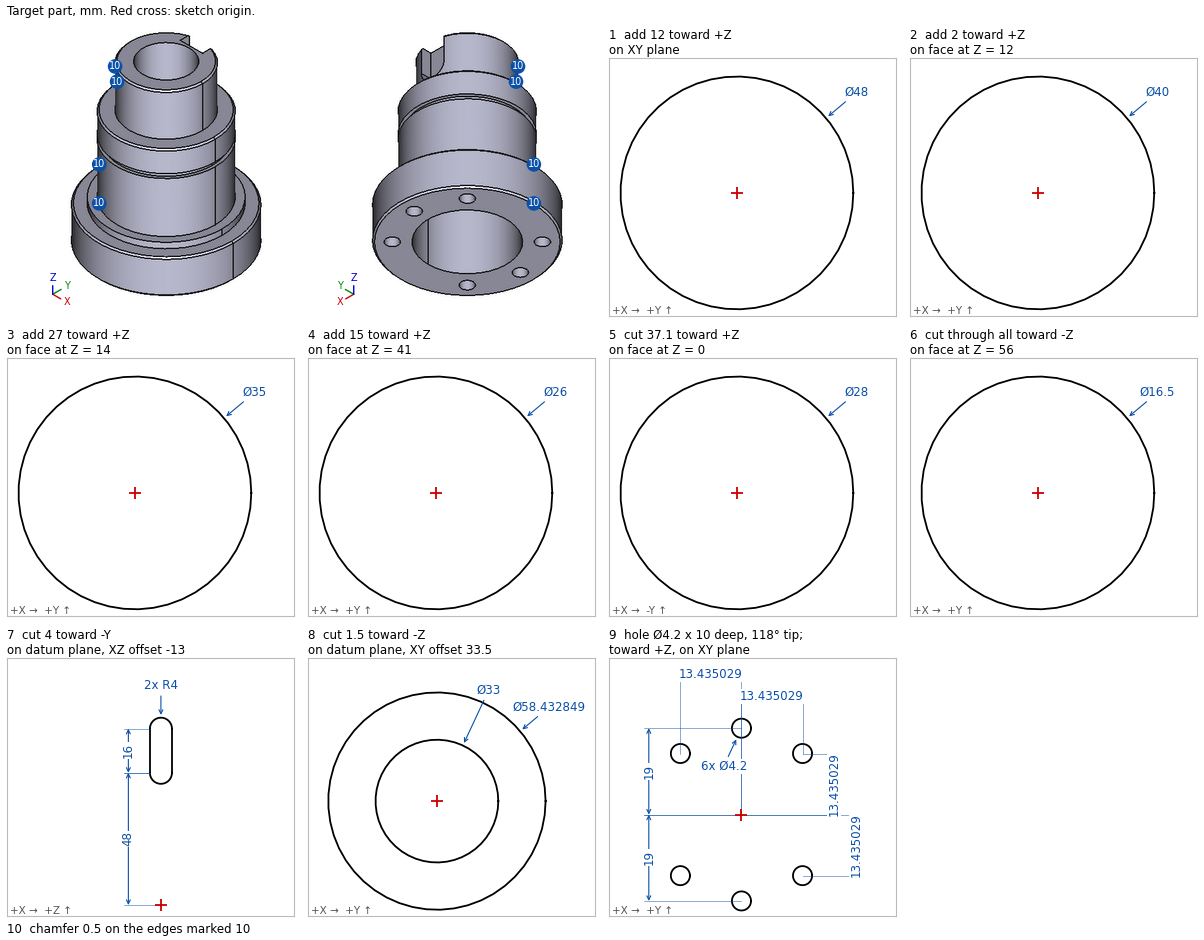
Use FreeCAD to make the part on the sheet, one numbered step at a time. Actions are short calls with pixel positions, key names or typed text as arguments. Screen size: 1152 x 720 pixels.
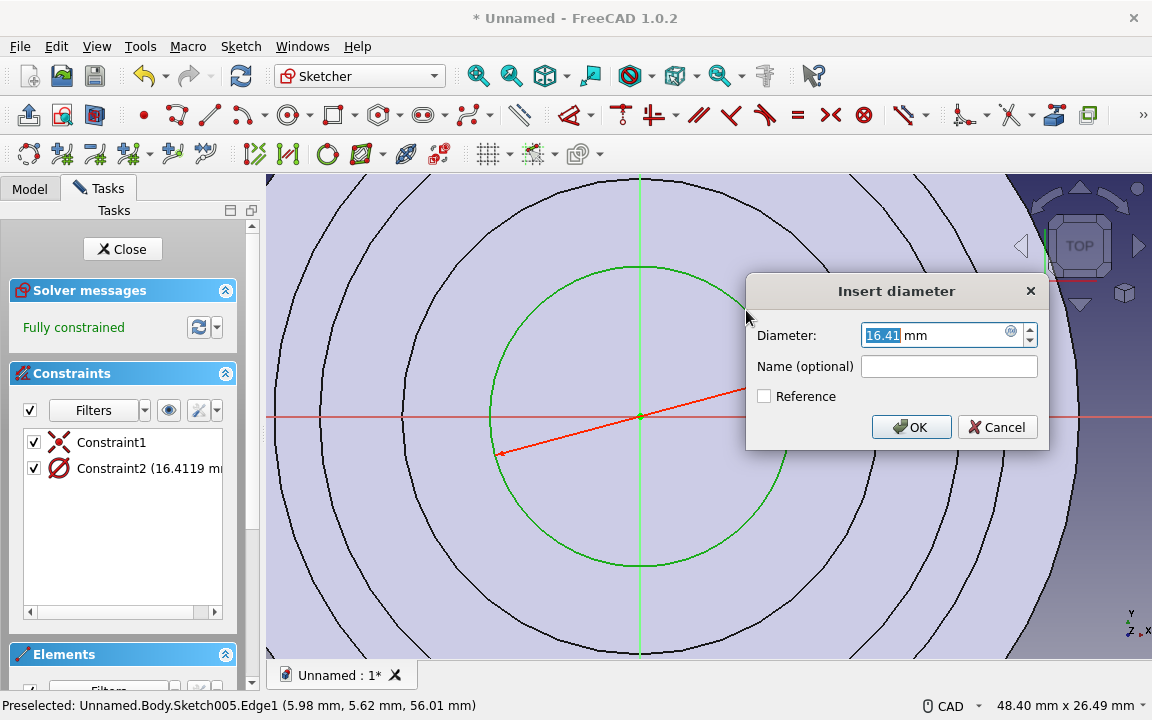
text(16.5)
key(Return)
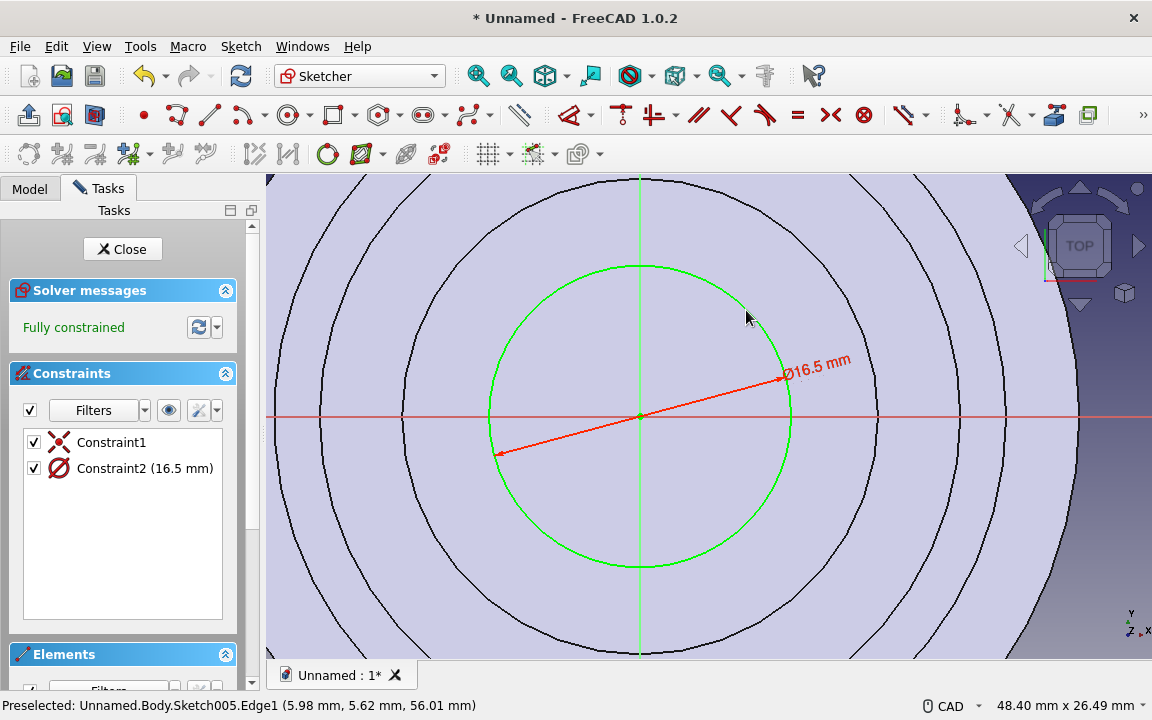
click(123, 249)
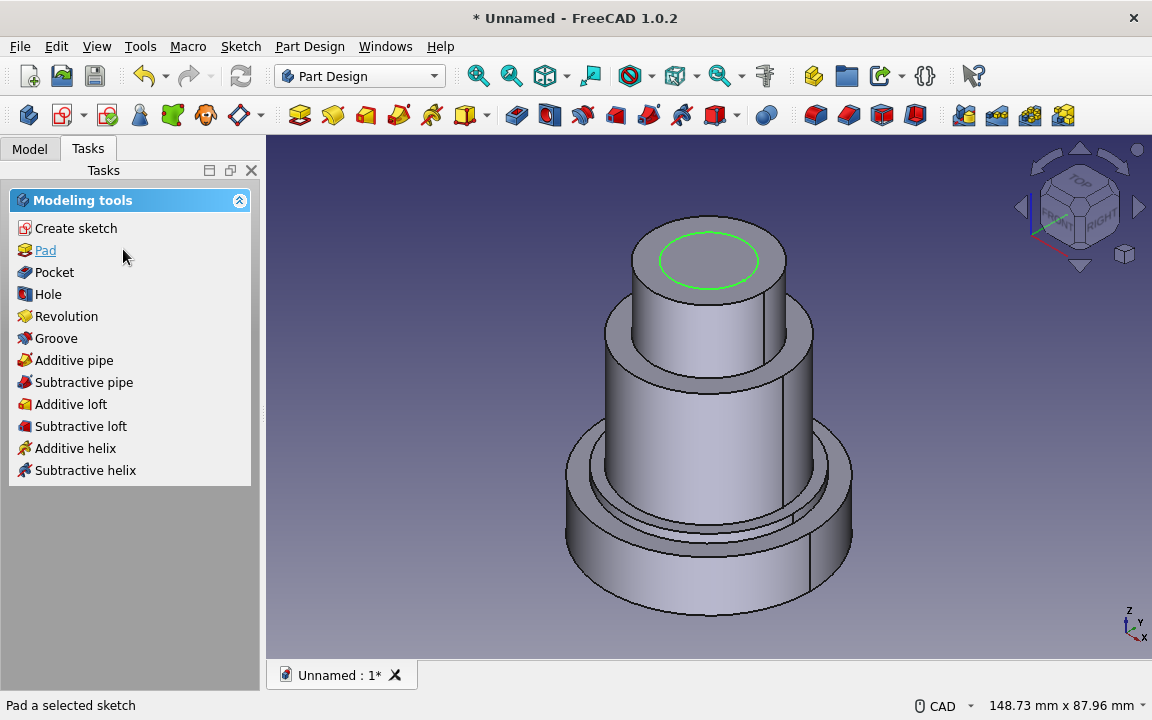
click(517, 116)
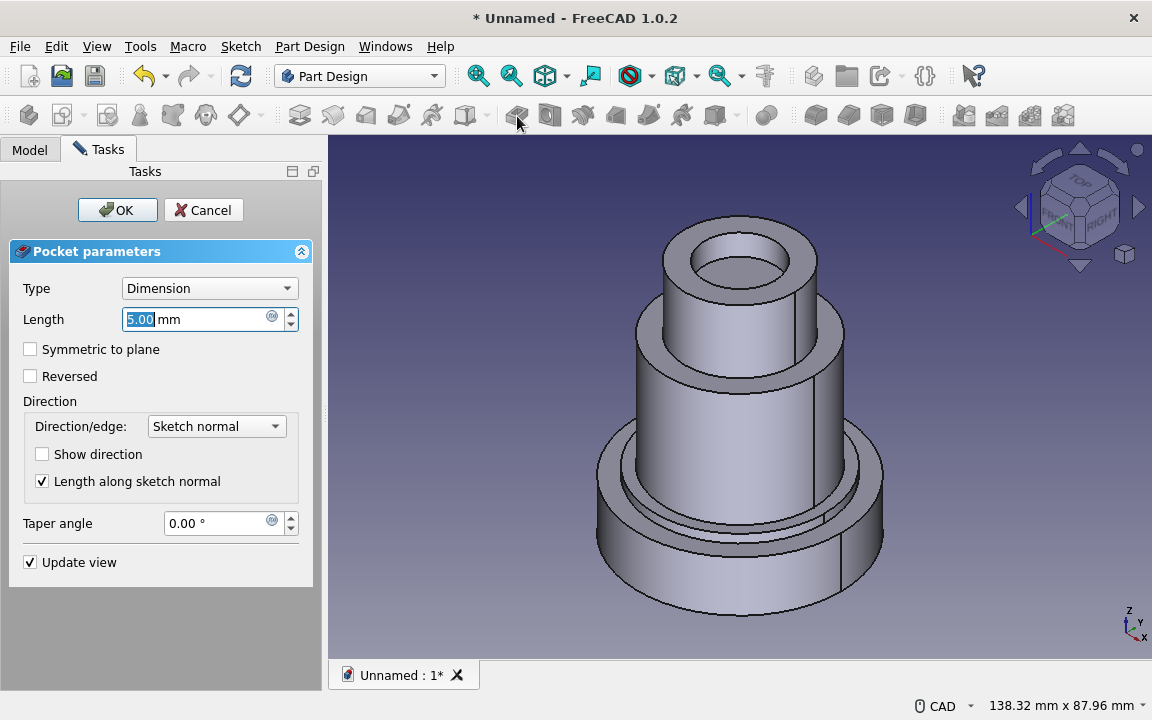
click(210, 288)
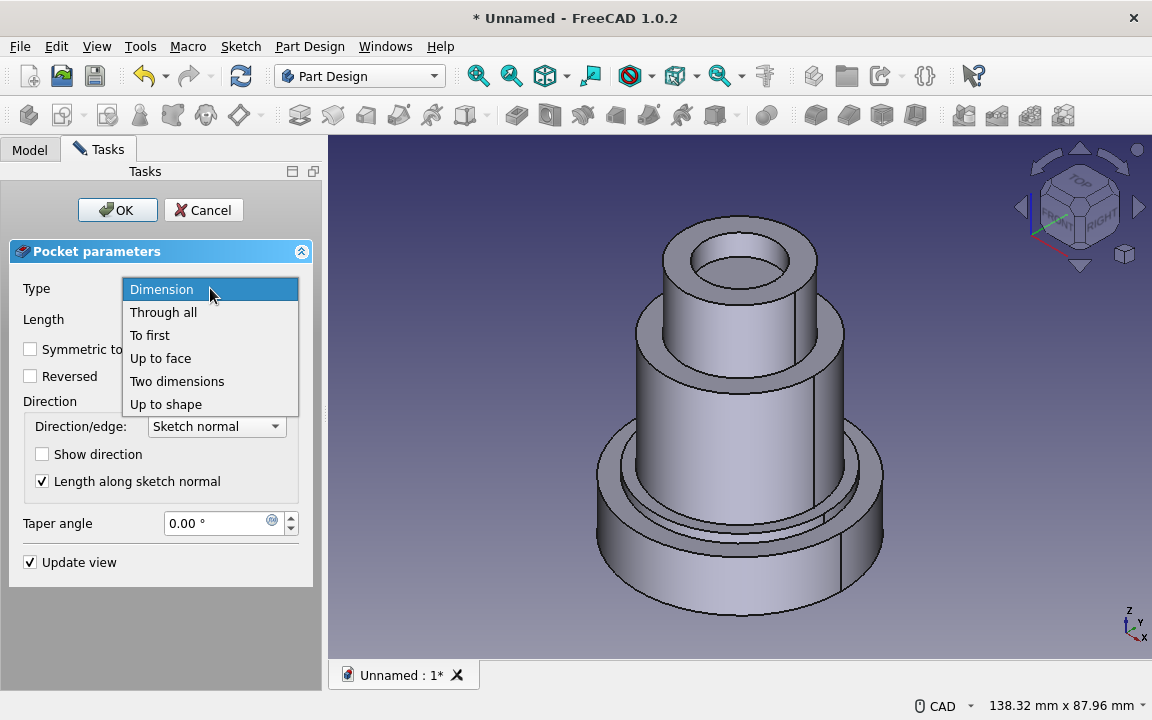
click(208, 312)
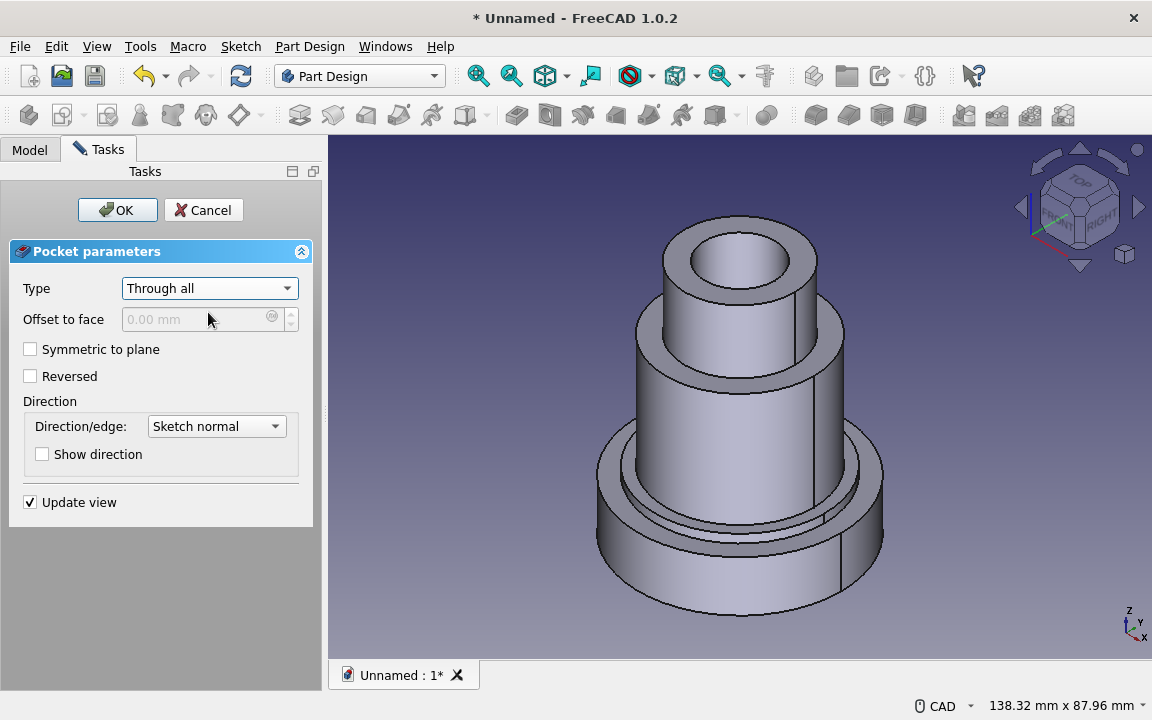
click(118, 210)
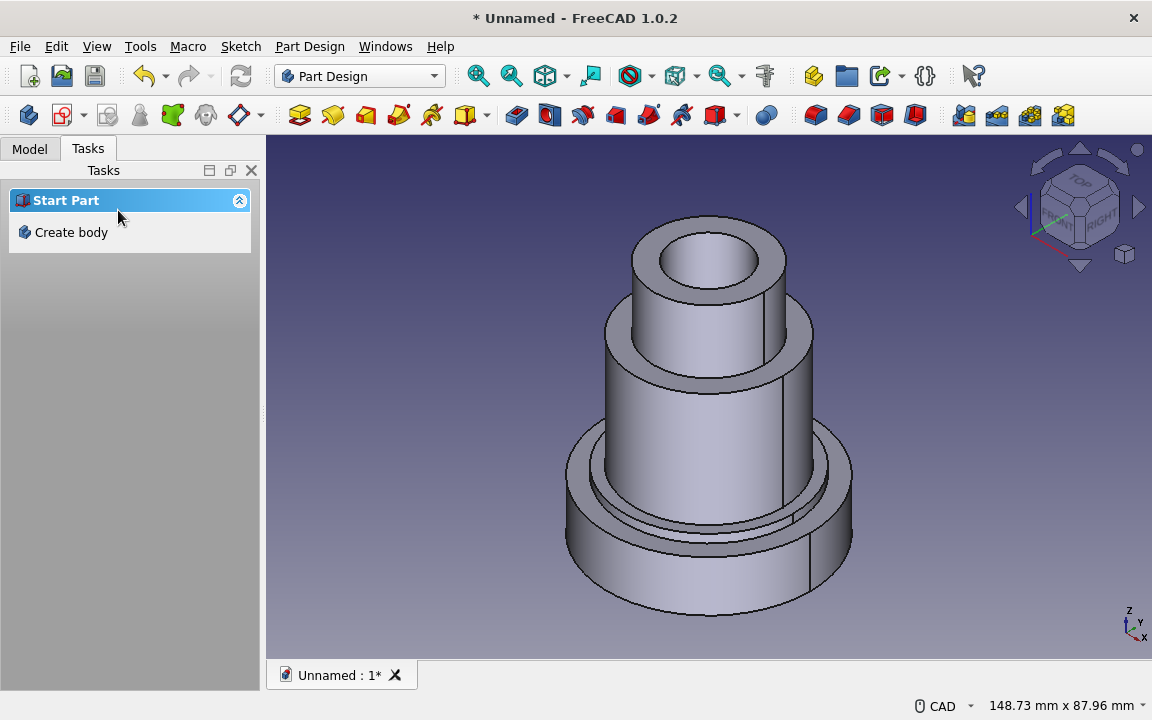
click(30, 148)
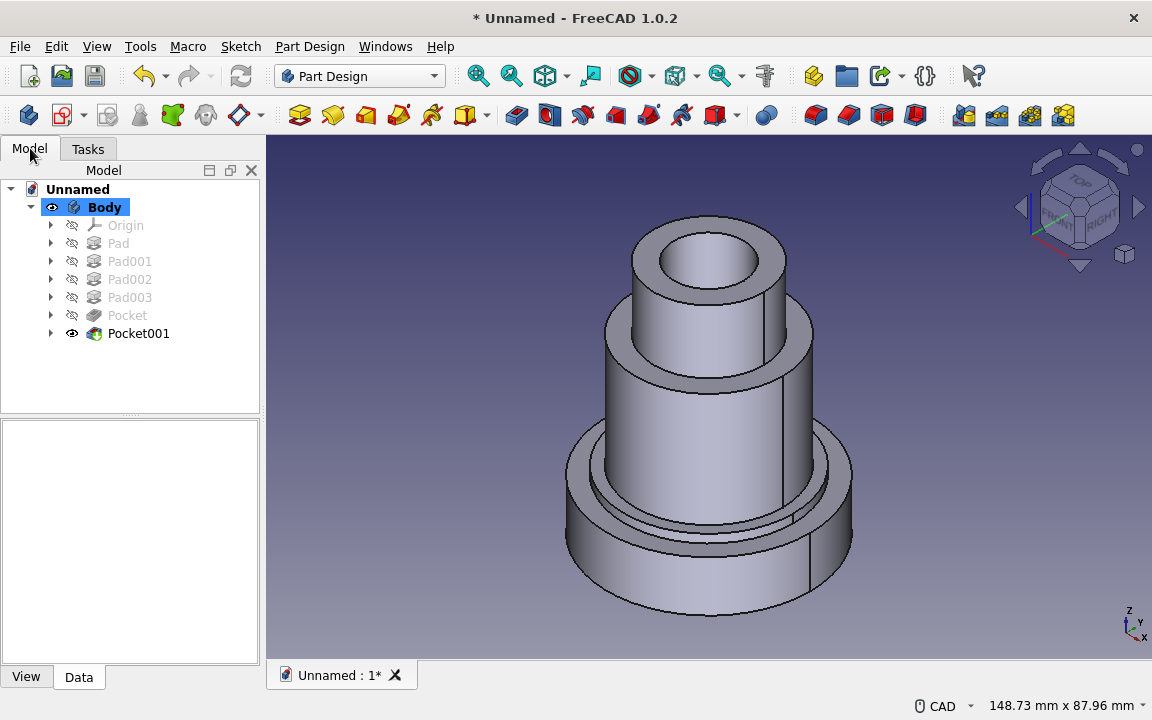
click(51, 225)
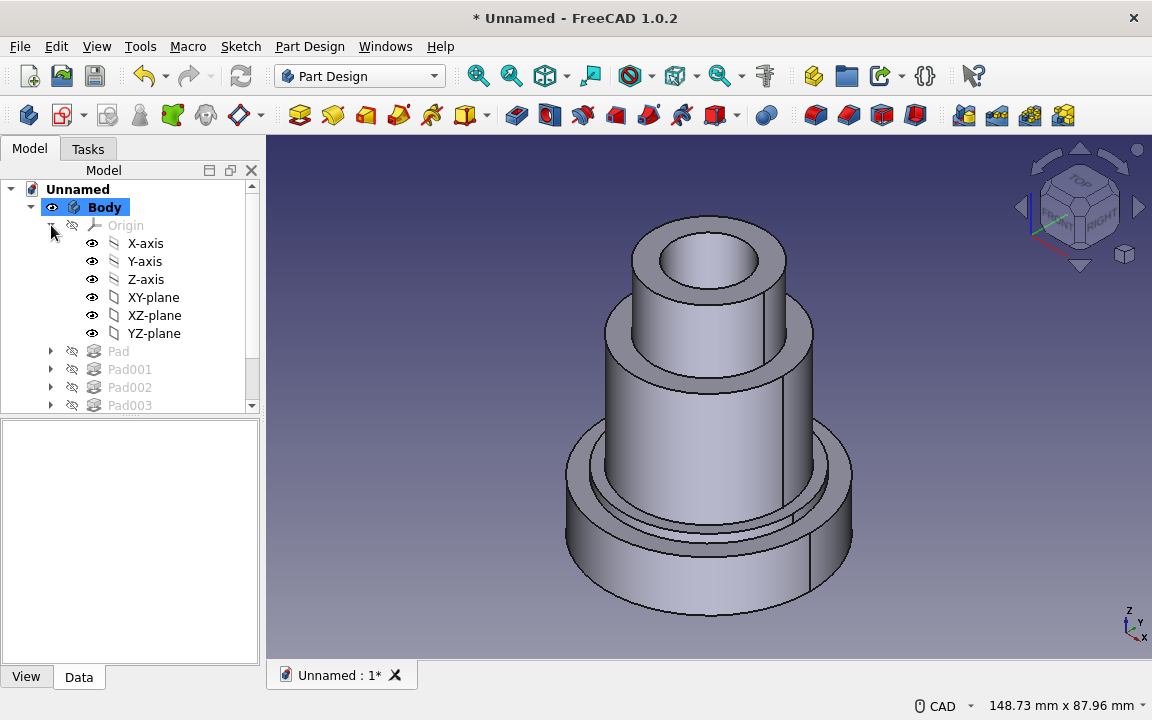
click(137, 315)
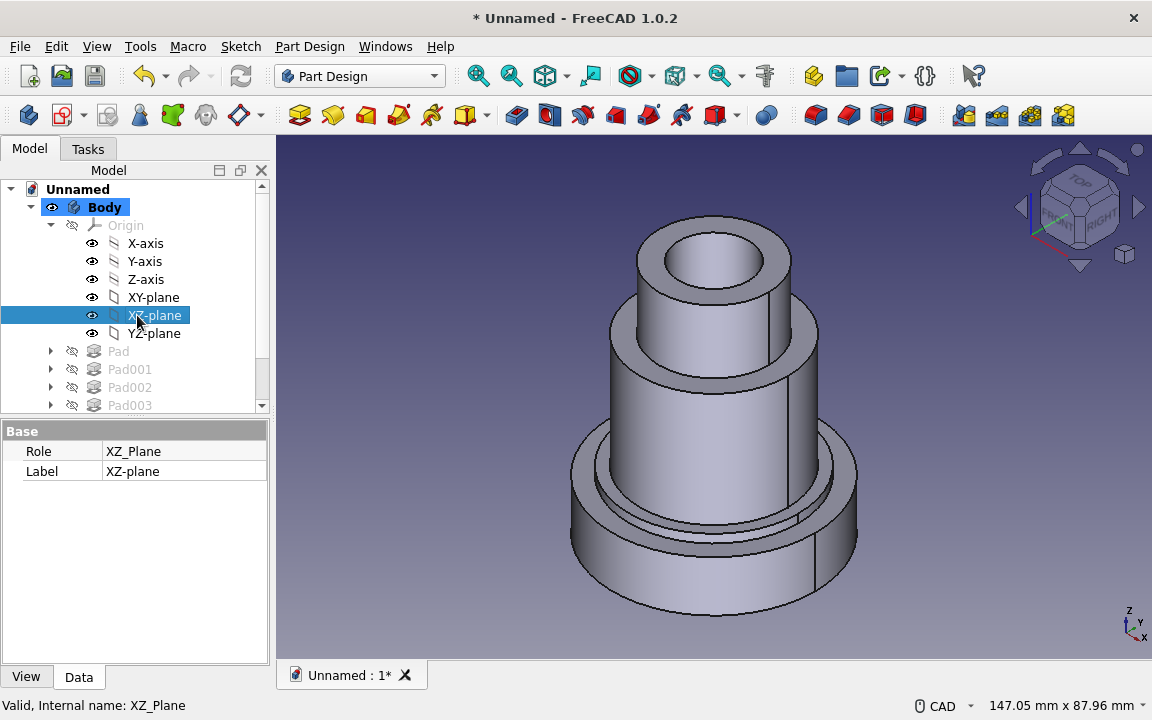
click(238, 116)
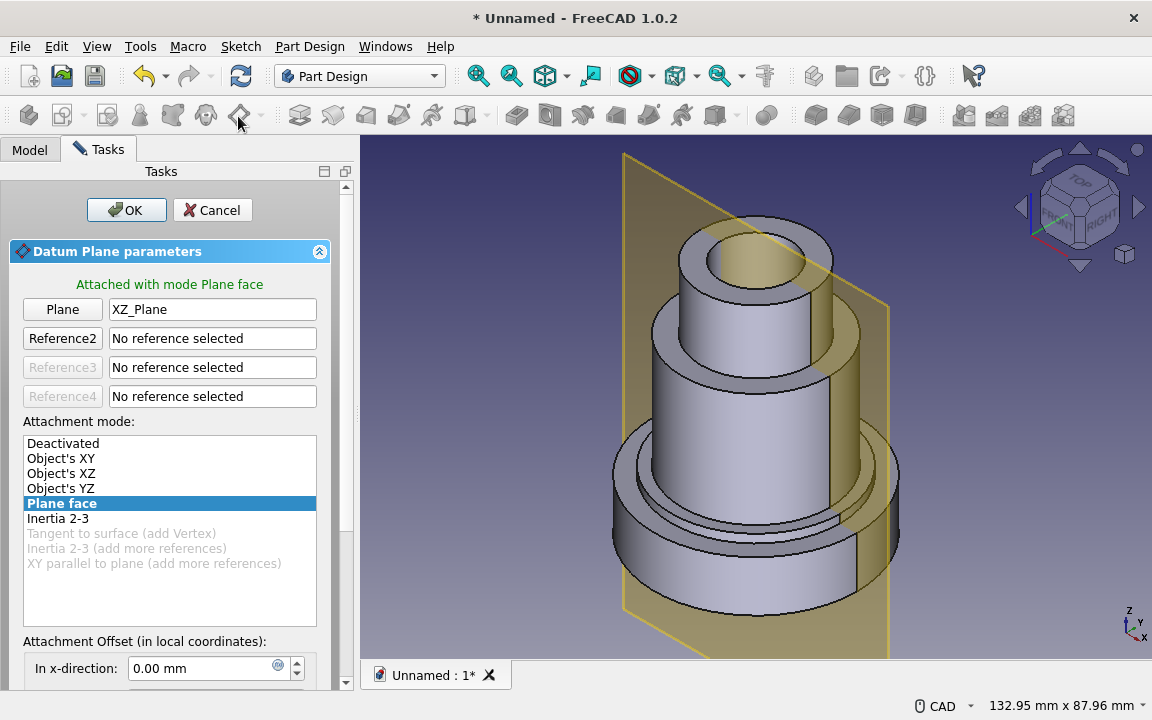
scroll(346, 436, down, 2)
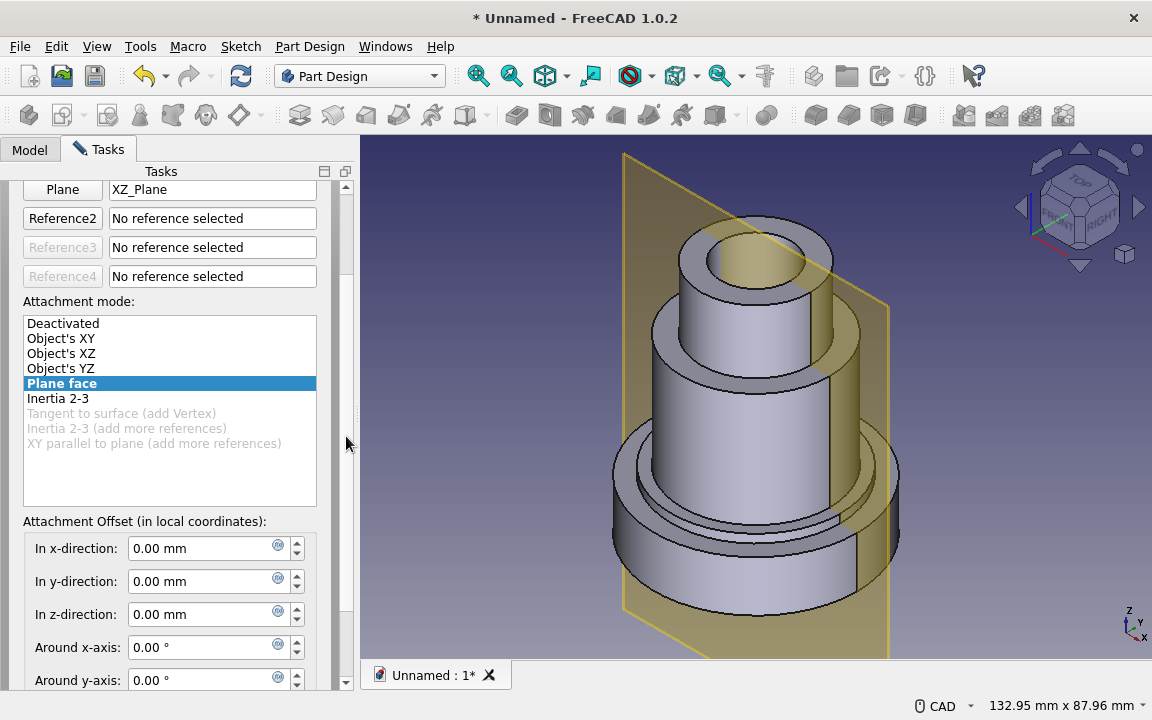
triple_click(210, 614)